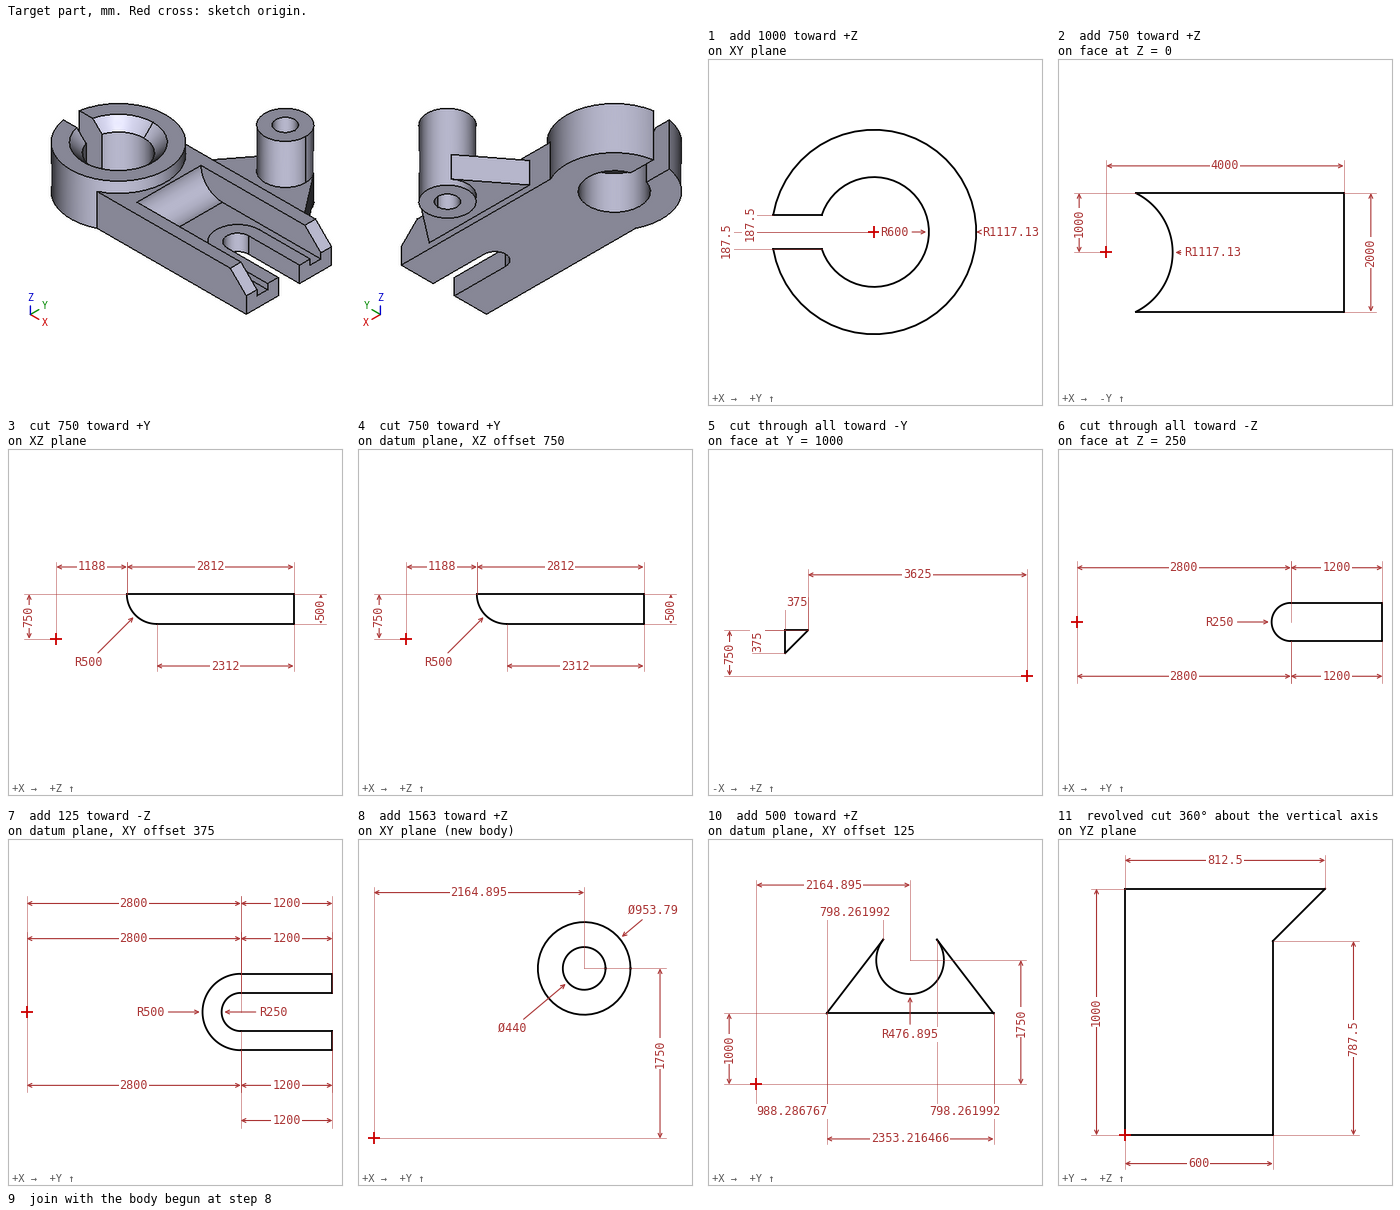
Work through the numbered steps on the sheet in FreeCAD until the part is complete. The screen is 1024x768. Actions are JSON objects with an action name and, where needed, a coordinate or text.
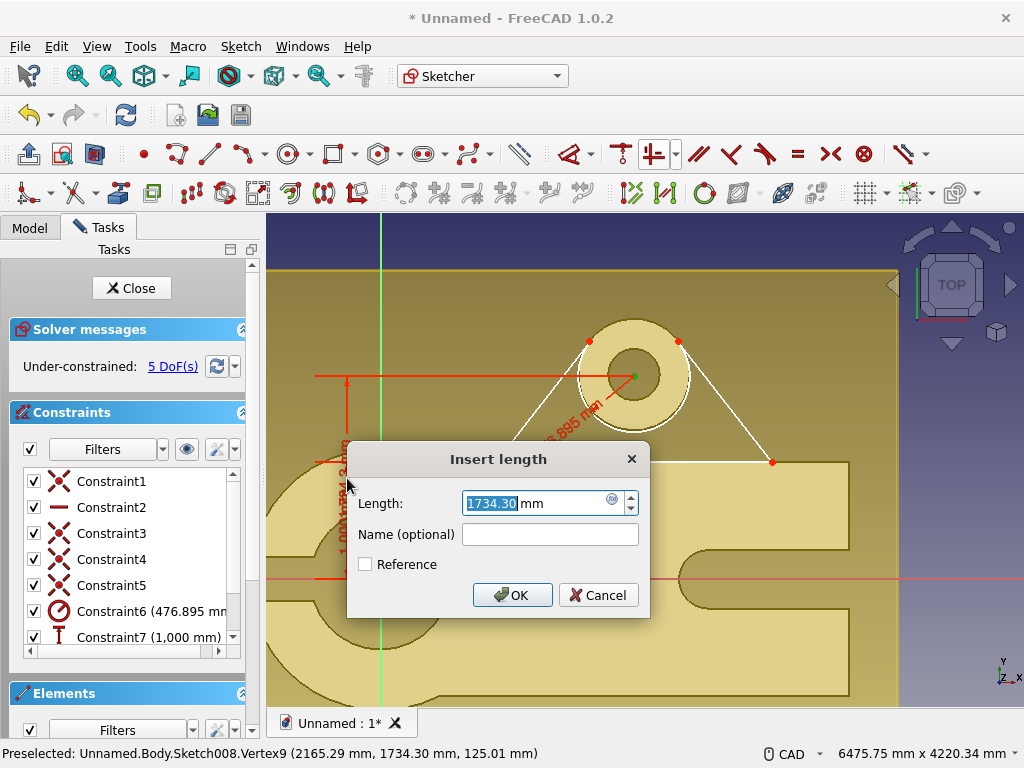
{"action": "type", "text": "1750"}
{"action": "key", "text": "Return"}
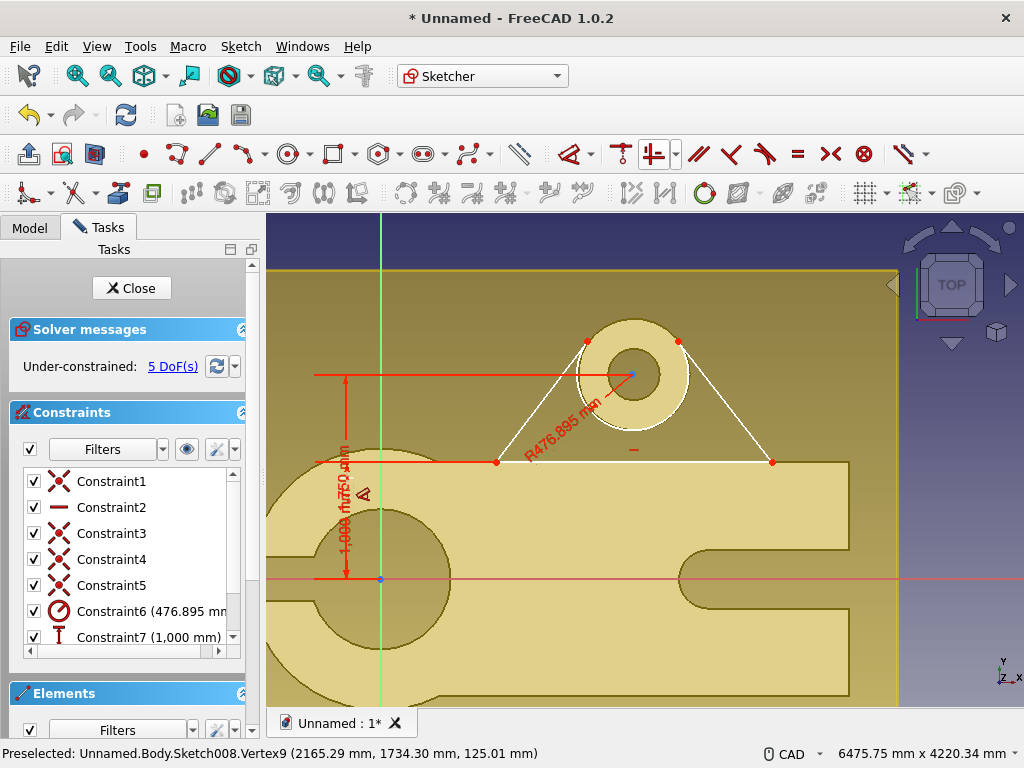
{"action": "left_click", "coordinate": [633, 375]}
{"action": "left_click", "coordinate": [507, 613]}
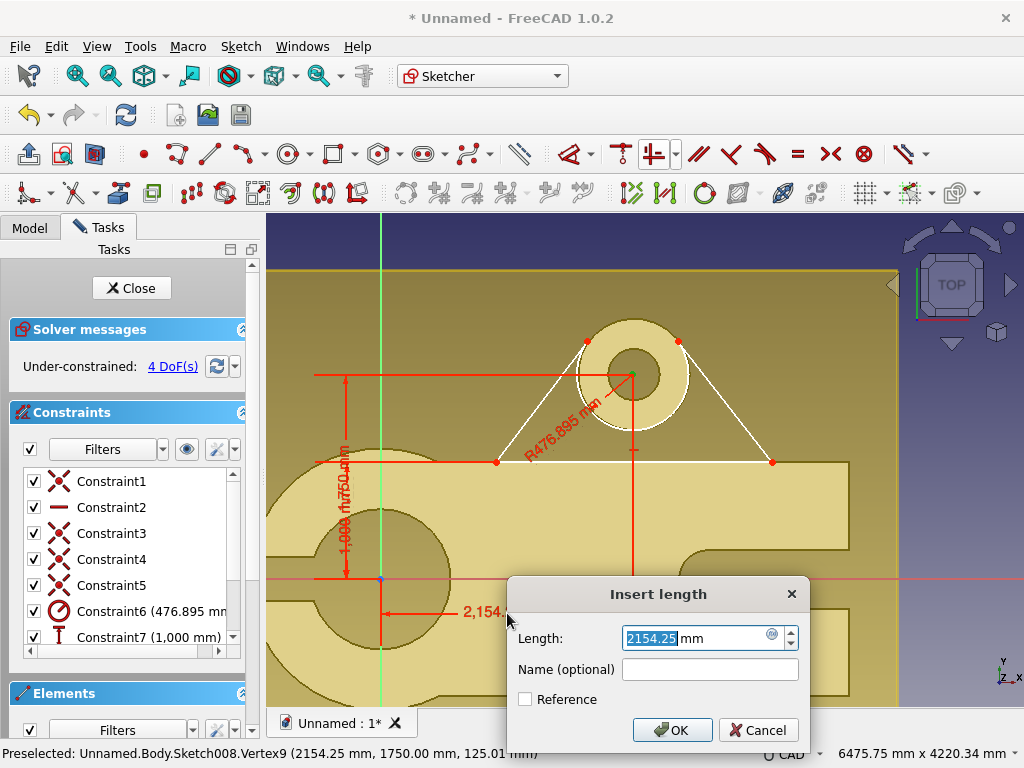
{"action": "type", "text": "2164.895"}
{"action": "key", "text": "Return"}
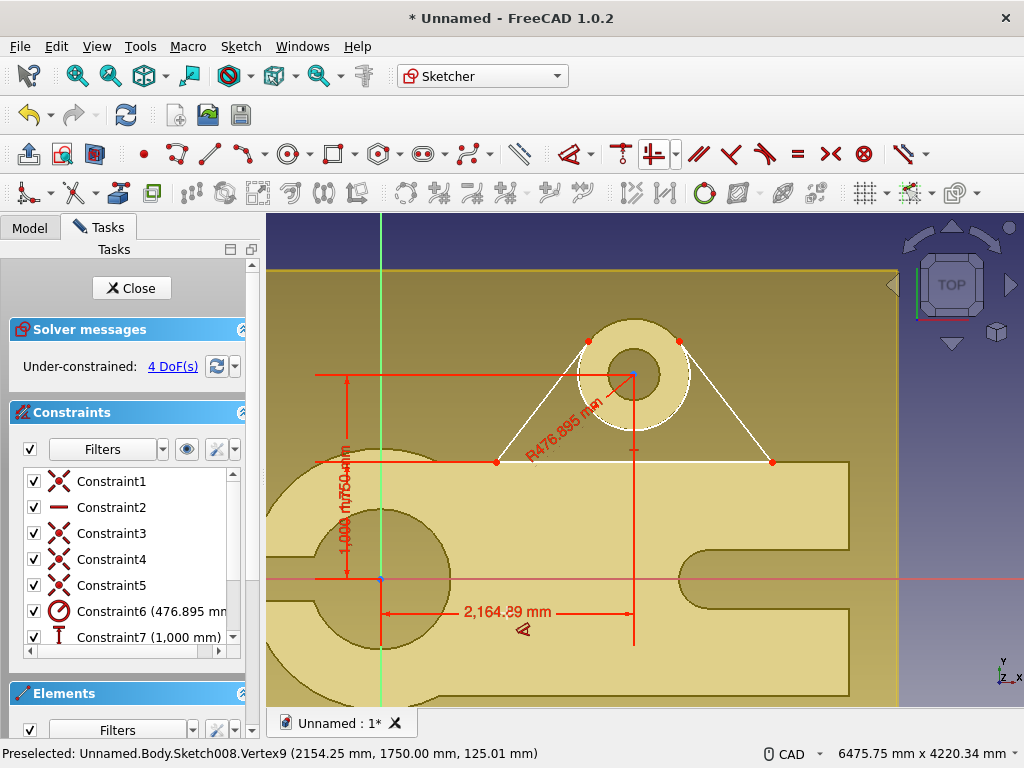
{"action": "left_click", "coordinate": [579, 462]}
{"action": "left_click", "coordinate": [634, 496]}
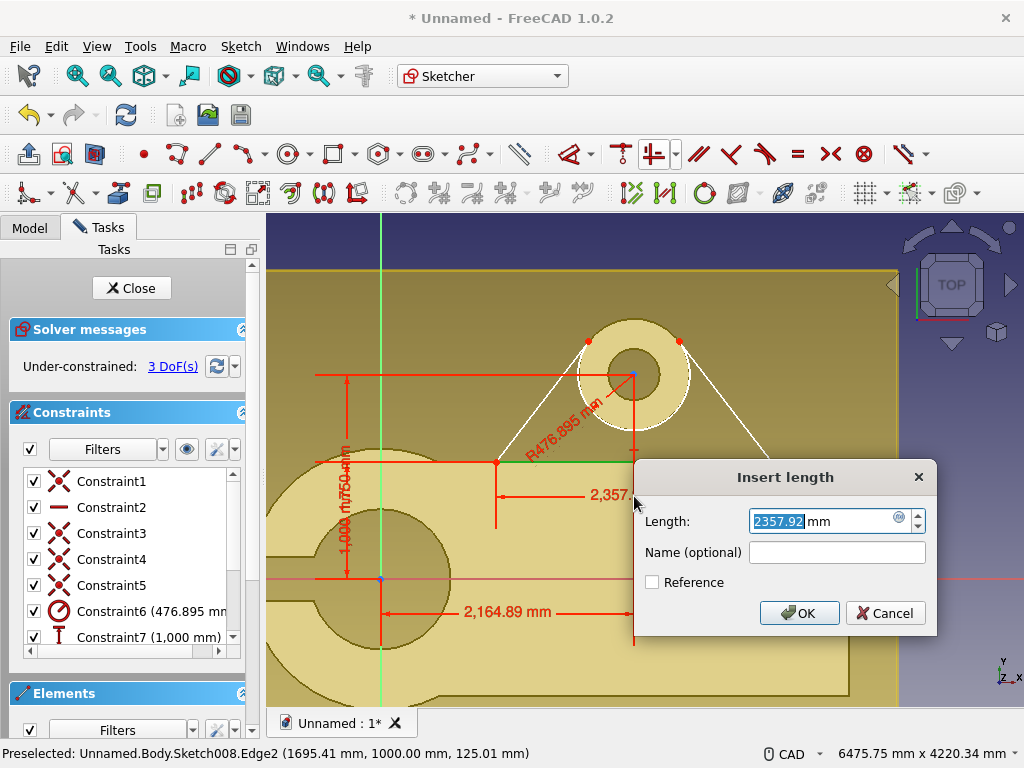
{"action": "type", "text": "2353.216466"}
{"action": "key", "text": "Return"}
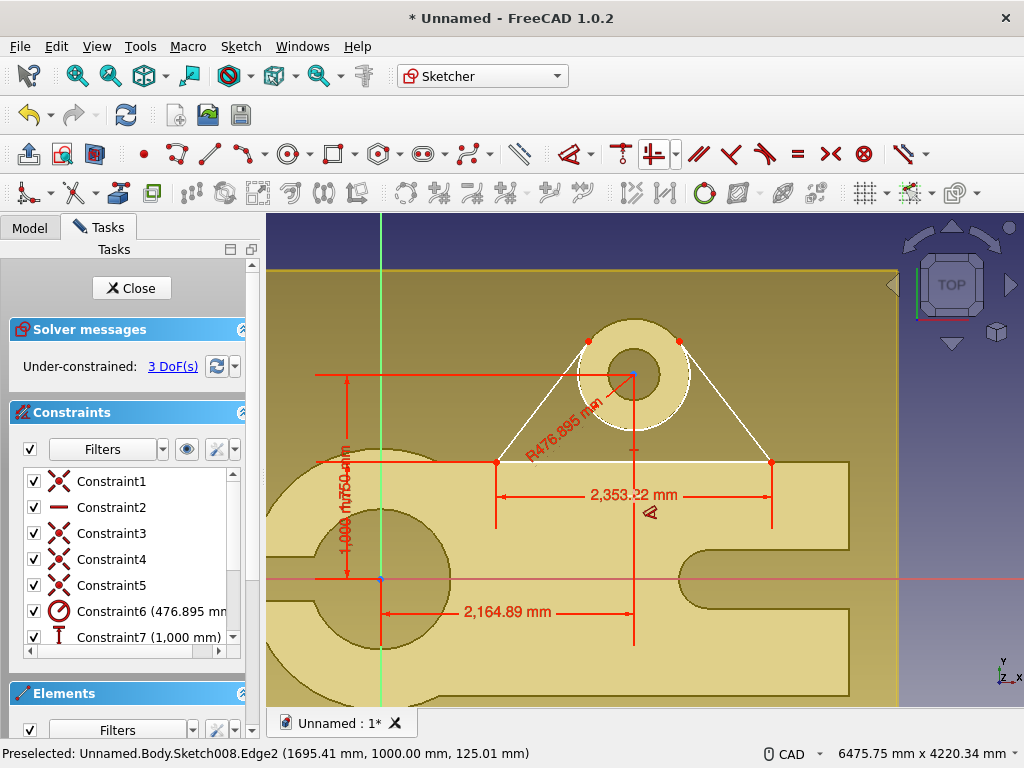
{"action": "left_click", "coordinate": [496, 462]}
{"action": "left_click", "coordinate": [412, 613]}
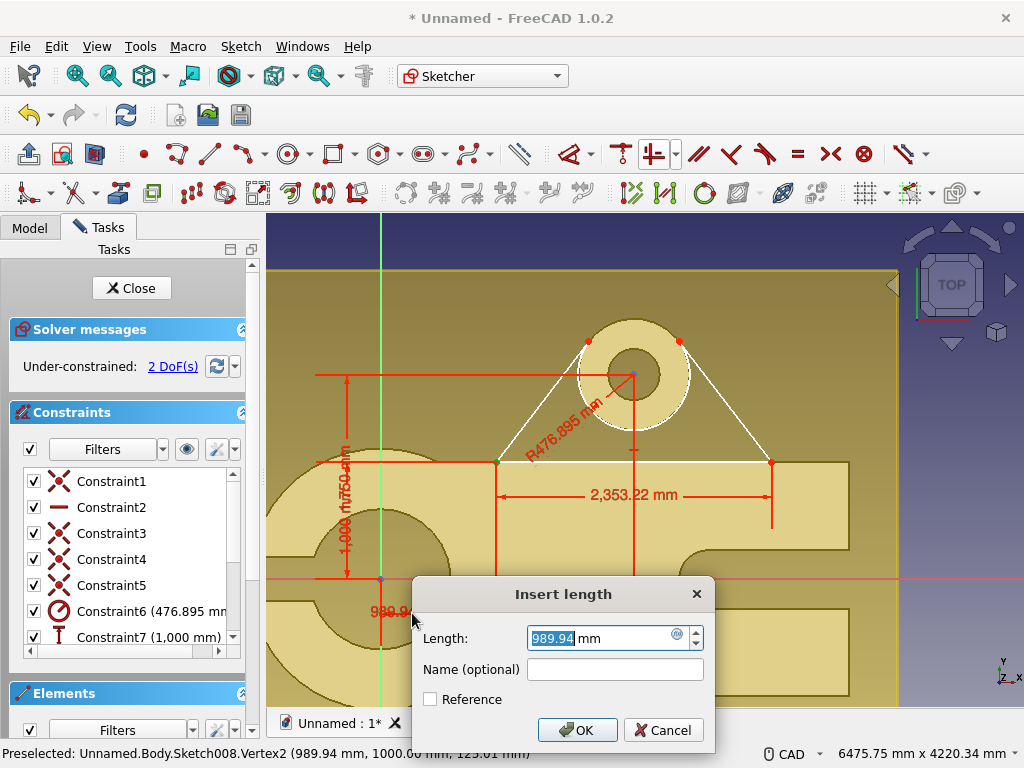
{"action": "type", "text": "988.286767"}
{"action": "key", "text": "Return"}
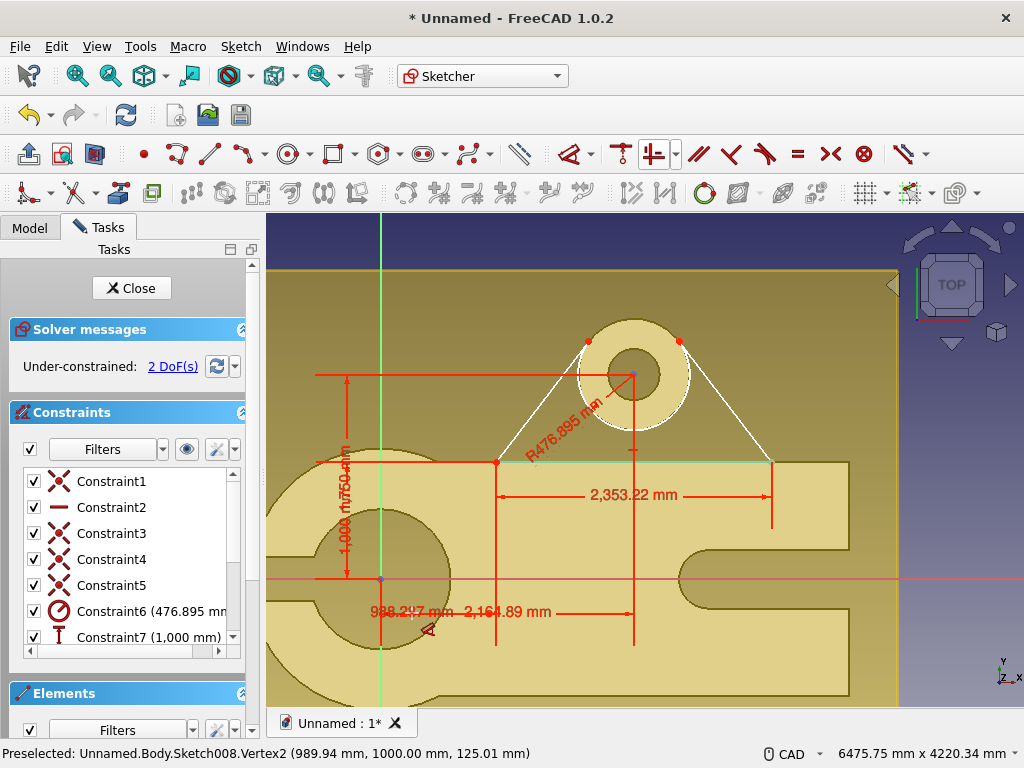
{"action": "left_click", "coordinate": [561, 378]}
{"action": "left_click", "coordinate": [542, 308]}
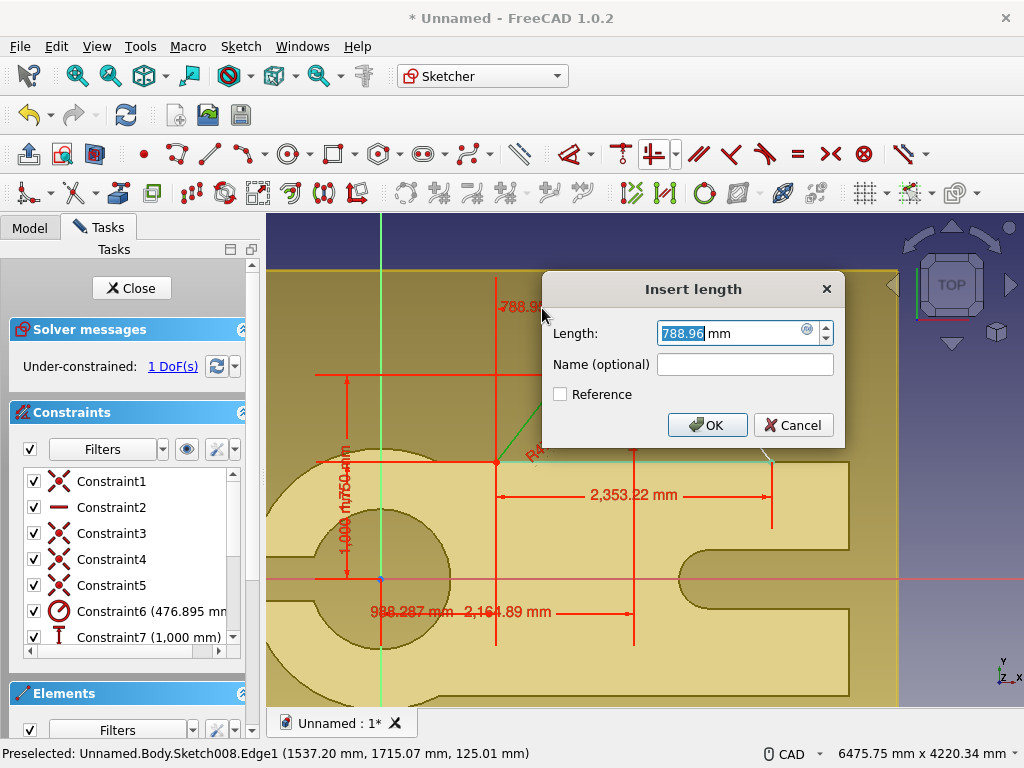
{"action": "type", "text": "798.261992"}
{"action": "key", "text": "Return"}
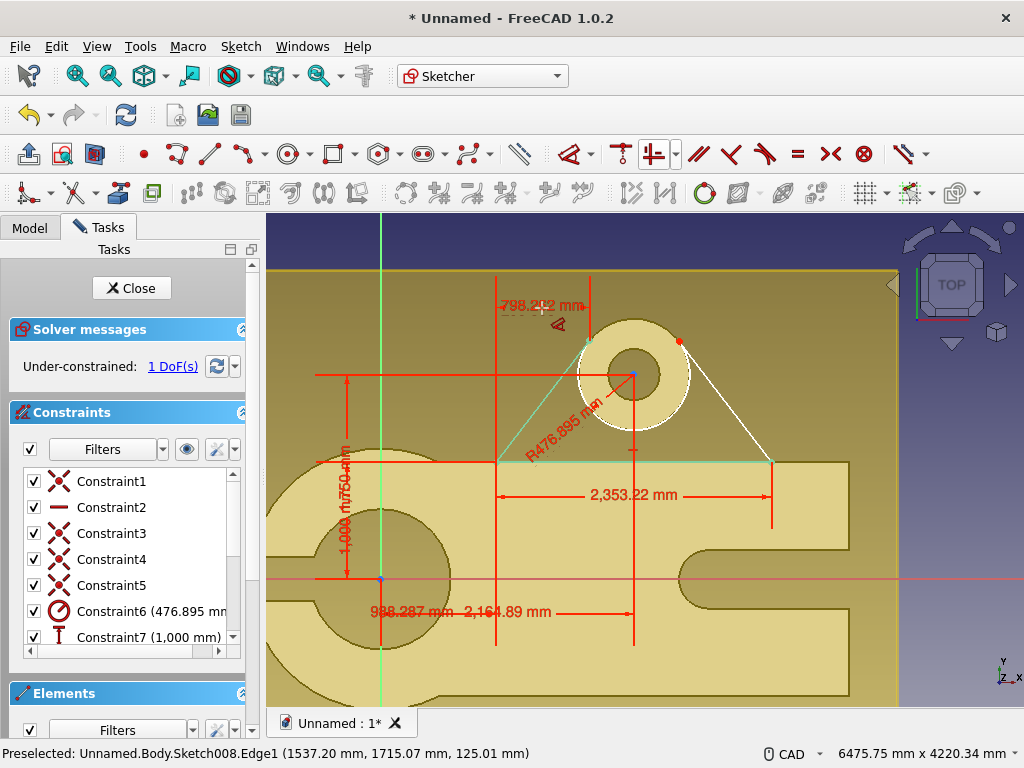
{"action": "left_click", "coordinate": [744, 426]}
{"action": "left_click", "coordinate": [726, 308]}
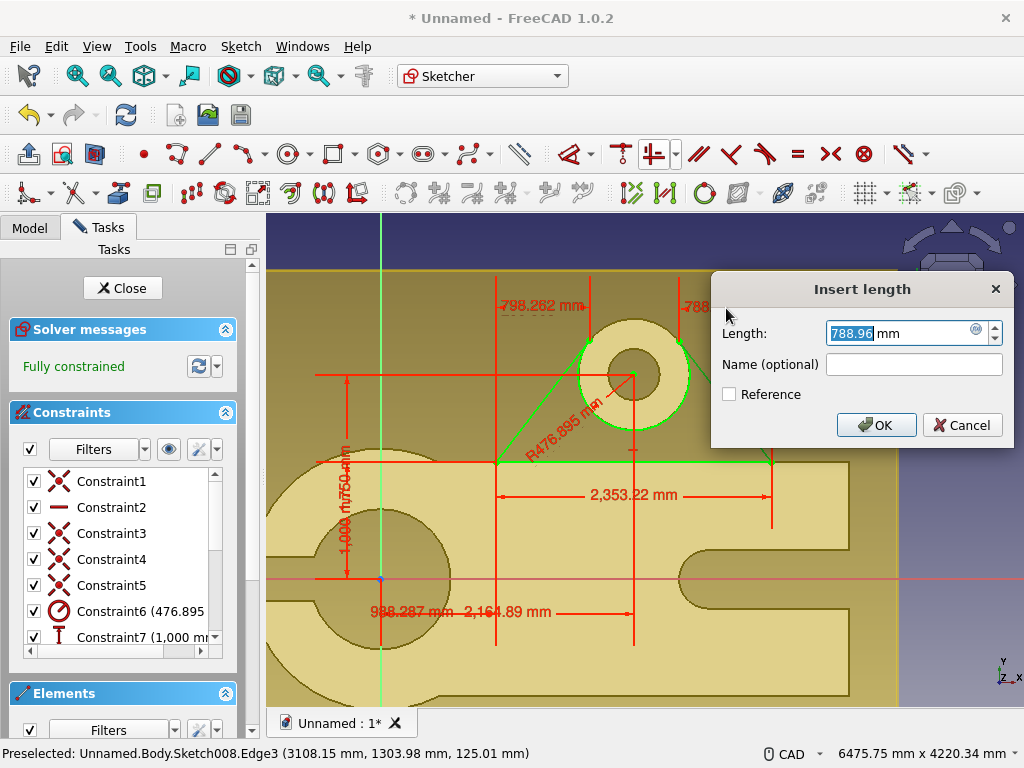
{"action": "type", "text": "798.261992"}
{"action": "key", "text": "Return"}
{"action": "key", "text": "Escape"}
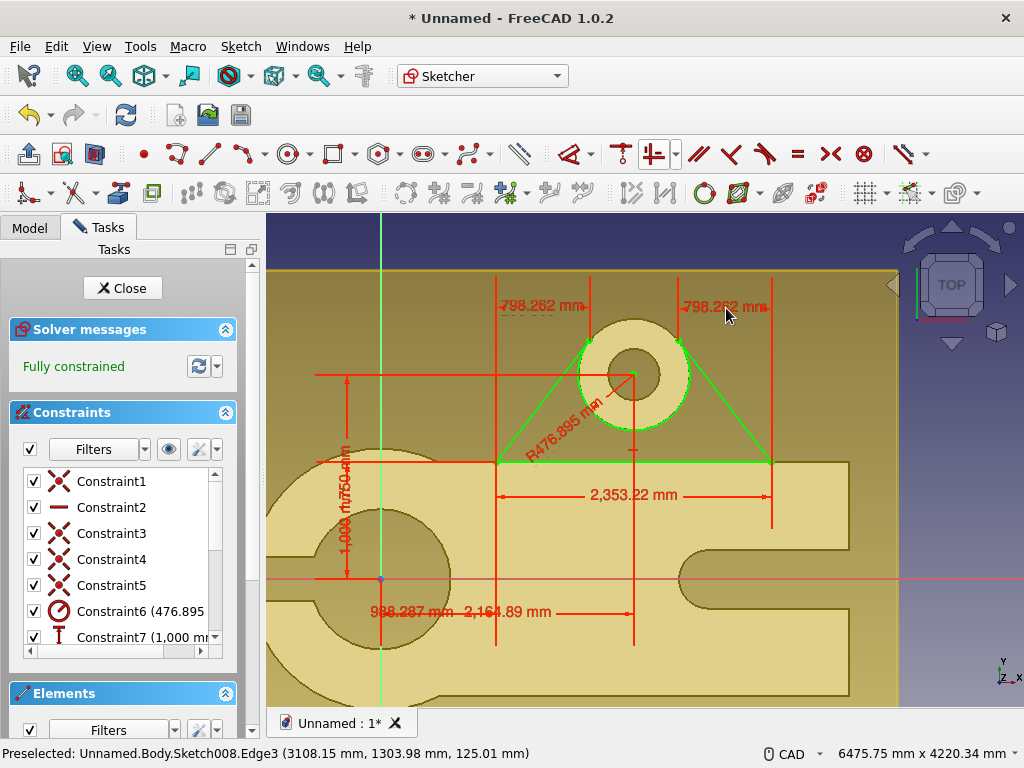
{"action": "left_click", "coordinate": [123, 288]}